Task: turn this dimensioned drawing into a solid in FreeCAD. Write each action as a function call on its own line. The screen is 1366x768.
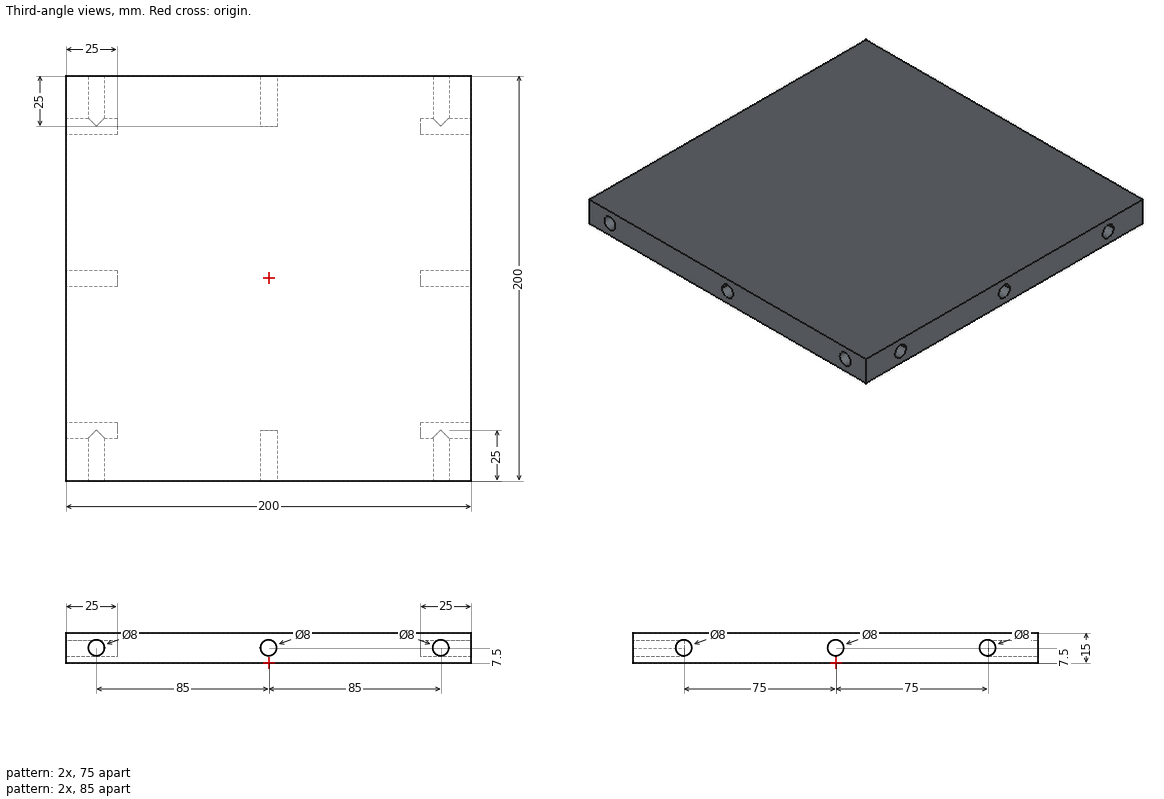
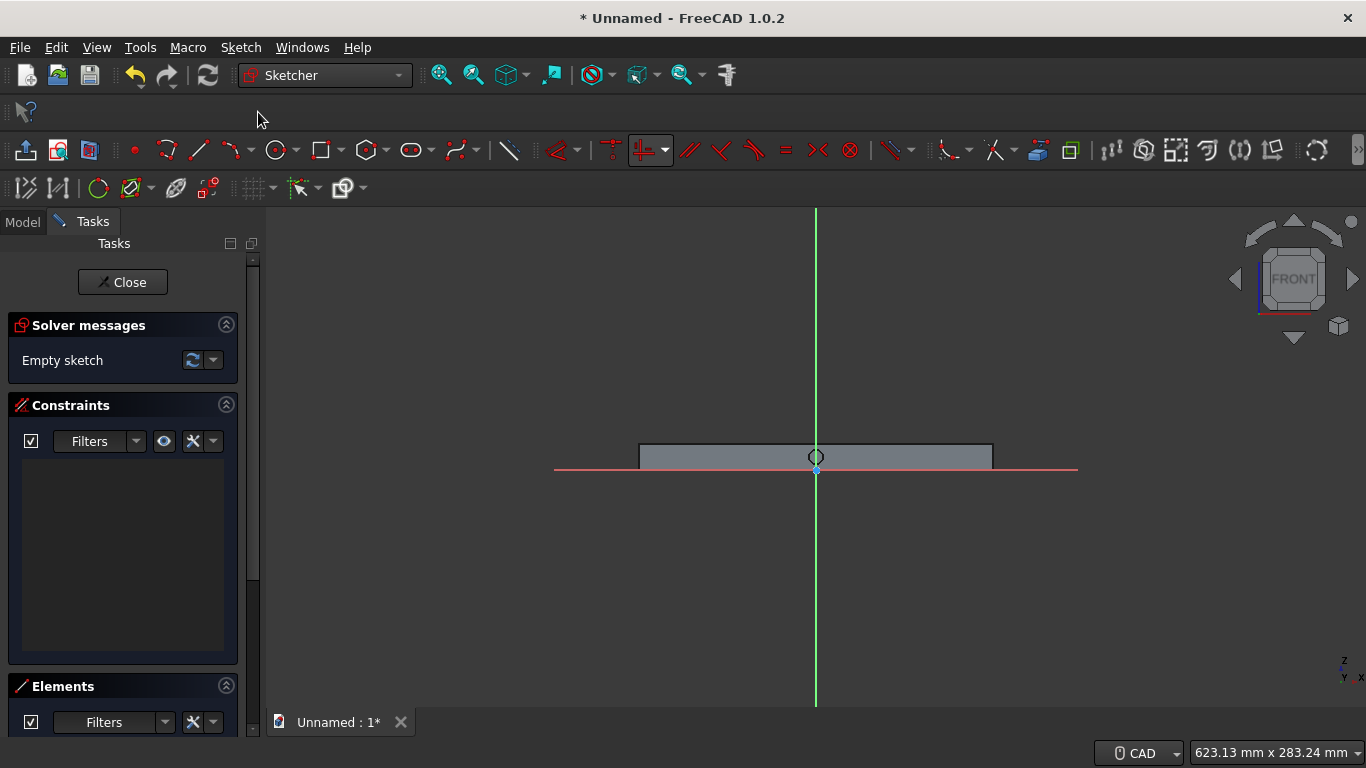
scroll(978, 457, up, 15)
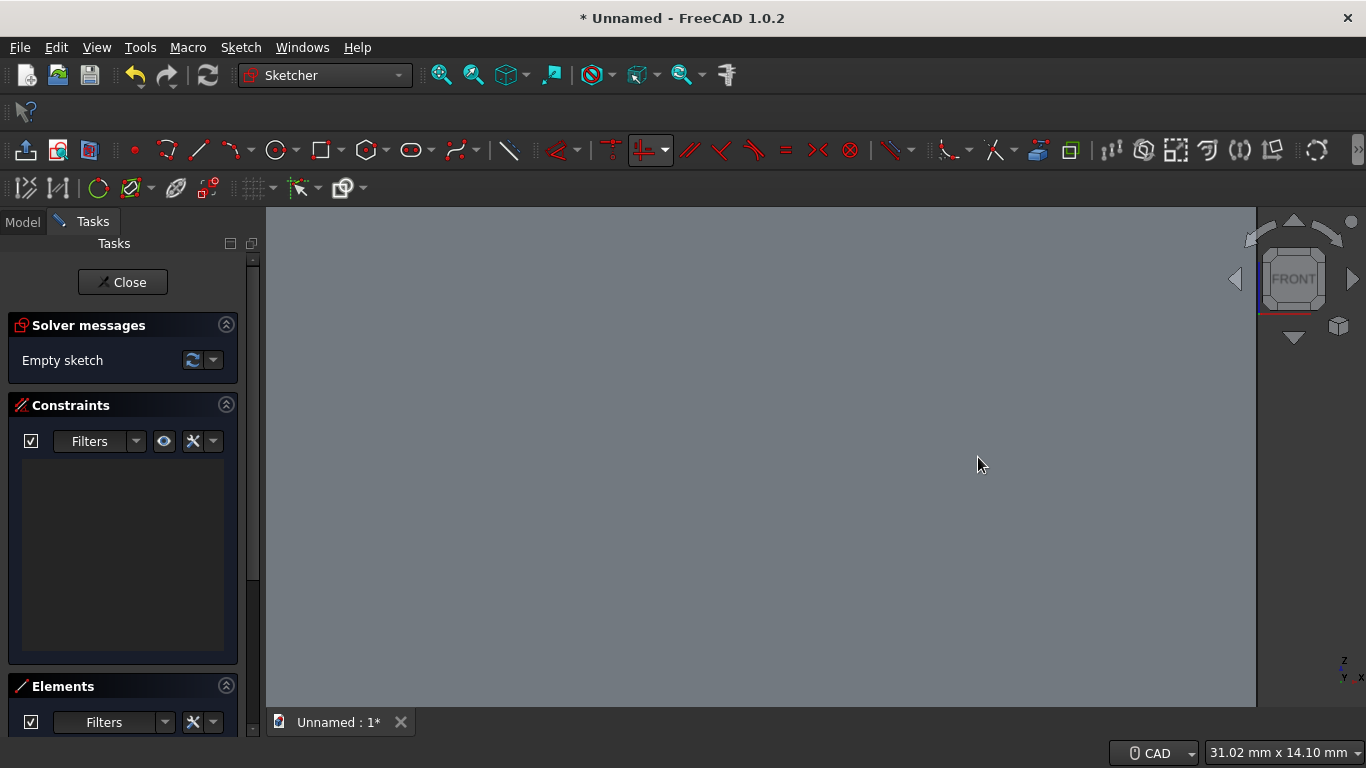
key(g)
key(c)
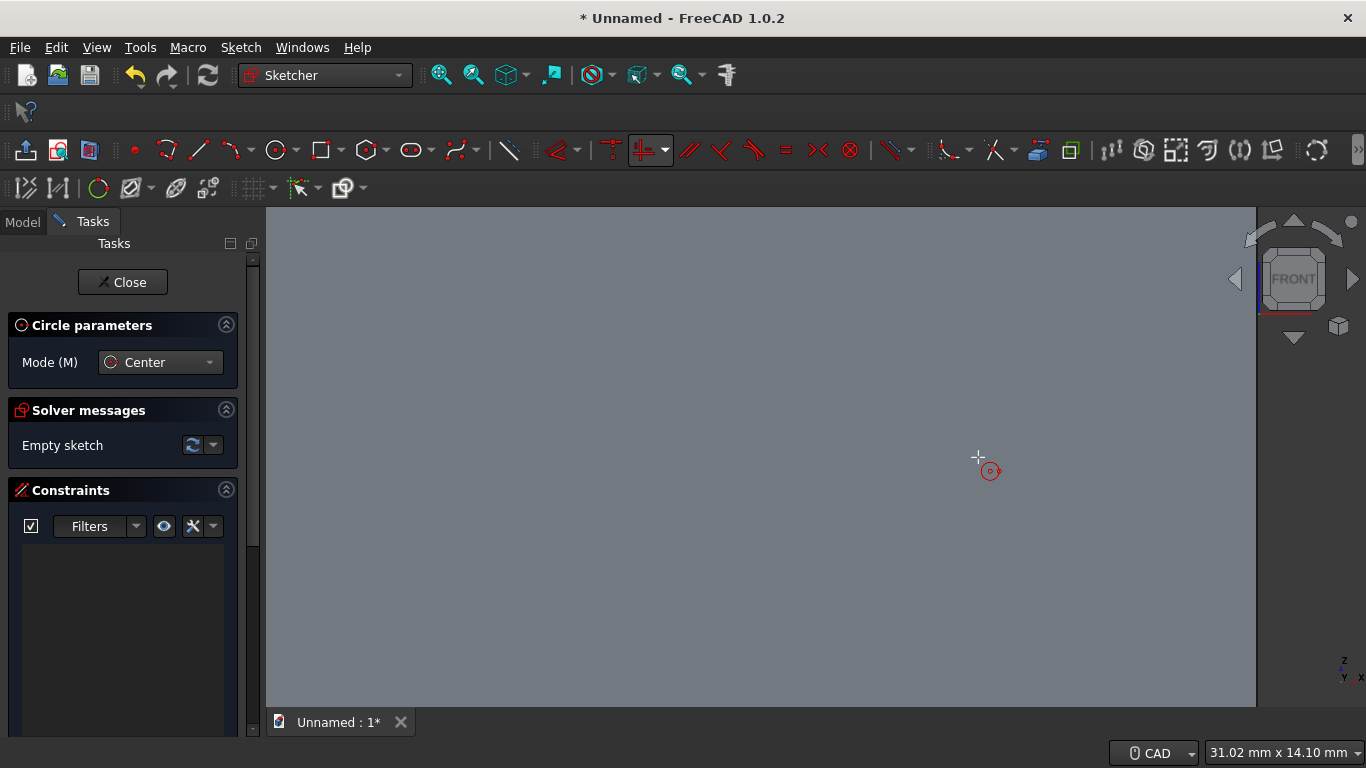
click(726, 447)
move(826, 347)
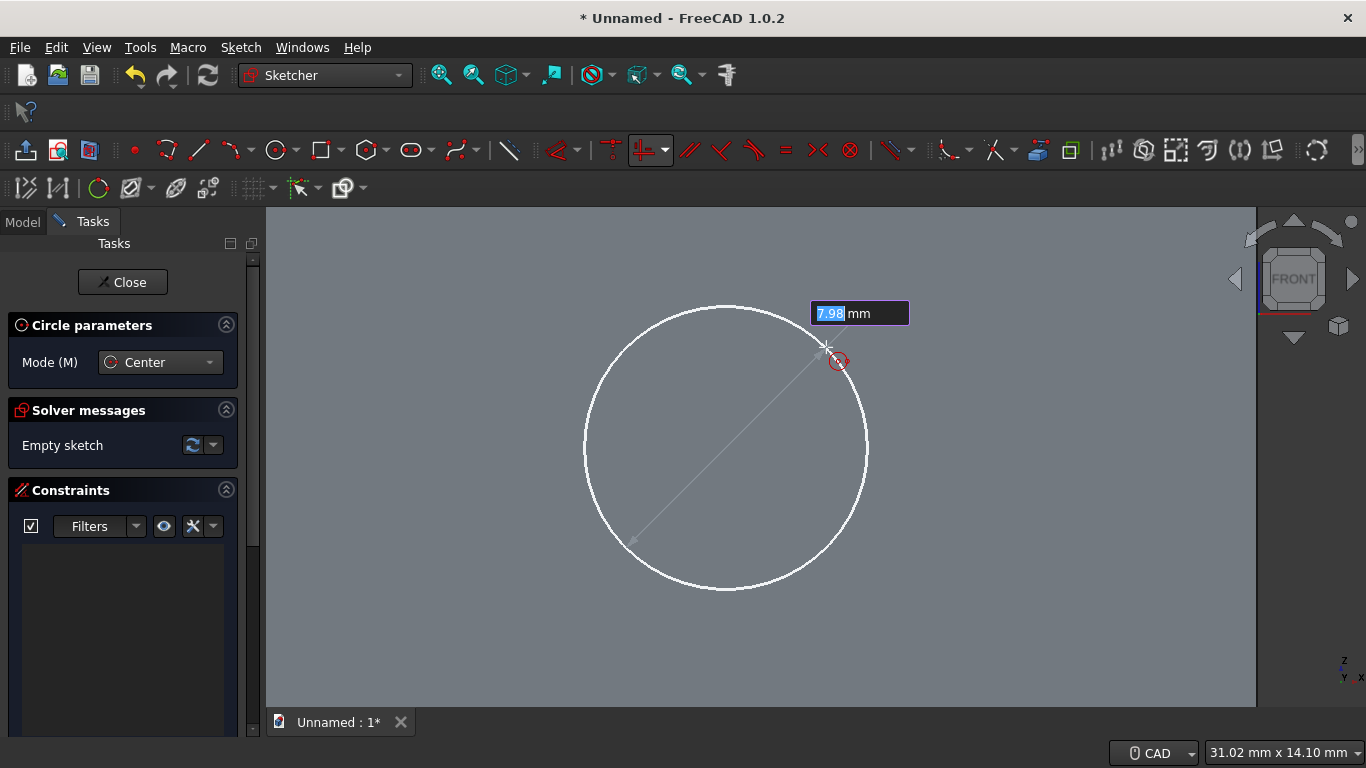
text(8)
key(Return)
key(Escape)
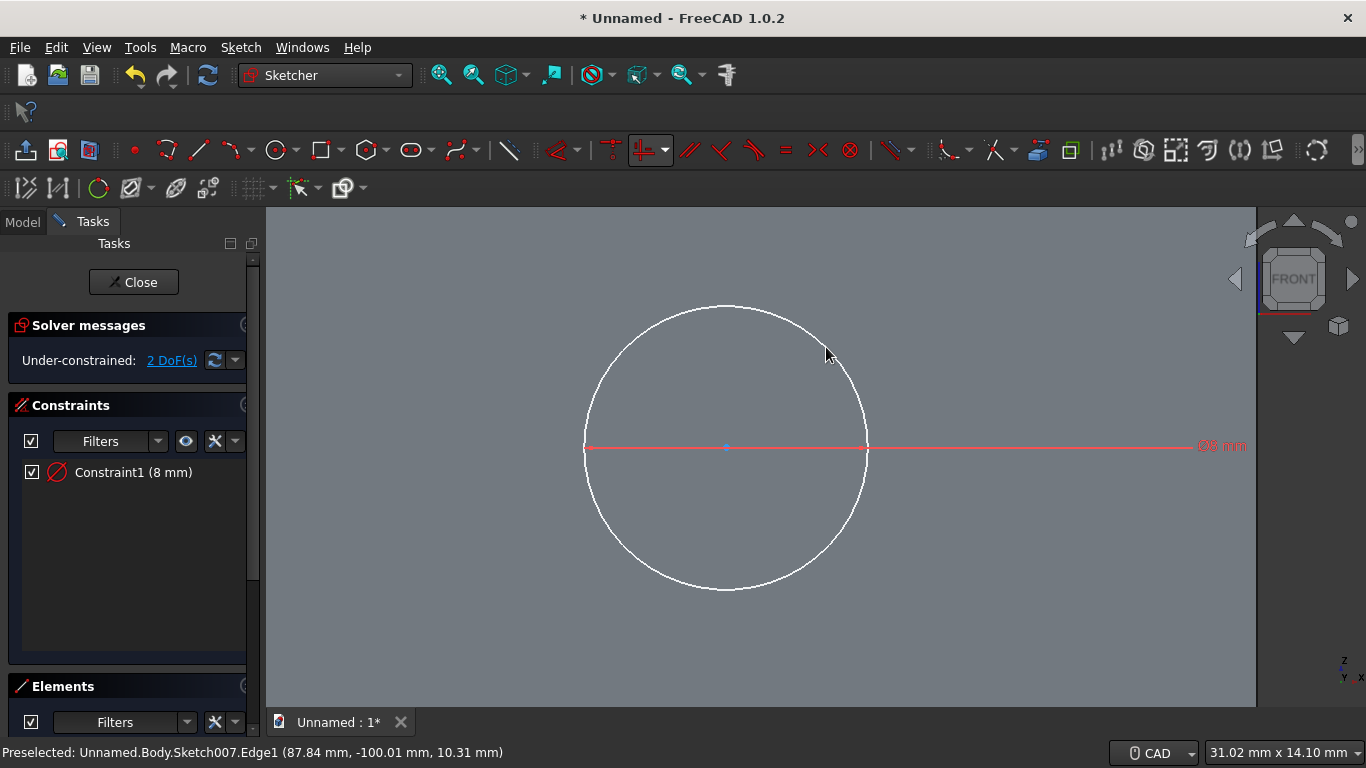
click(556, 150)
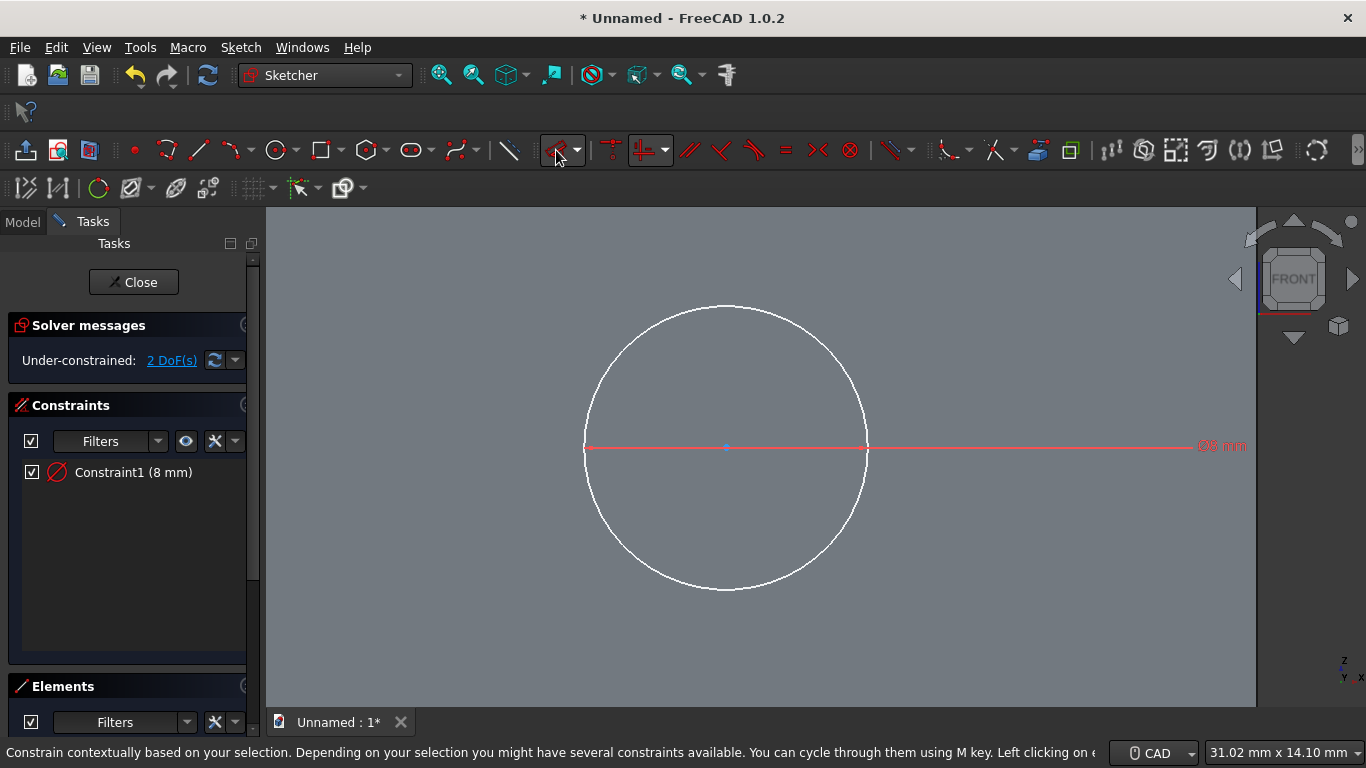
click(726, 448)
click(510, 414)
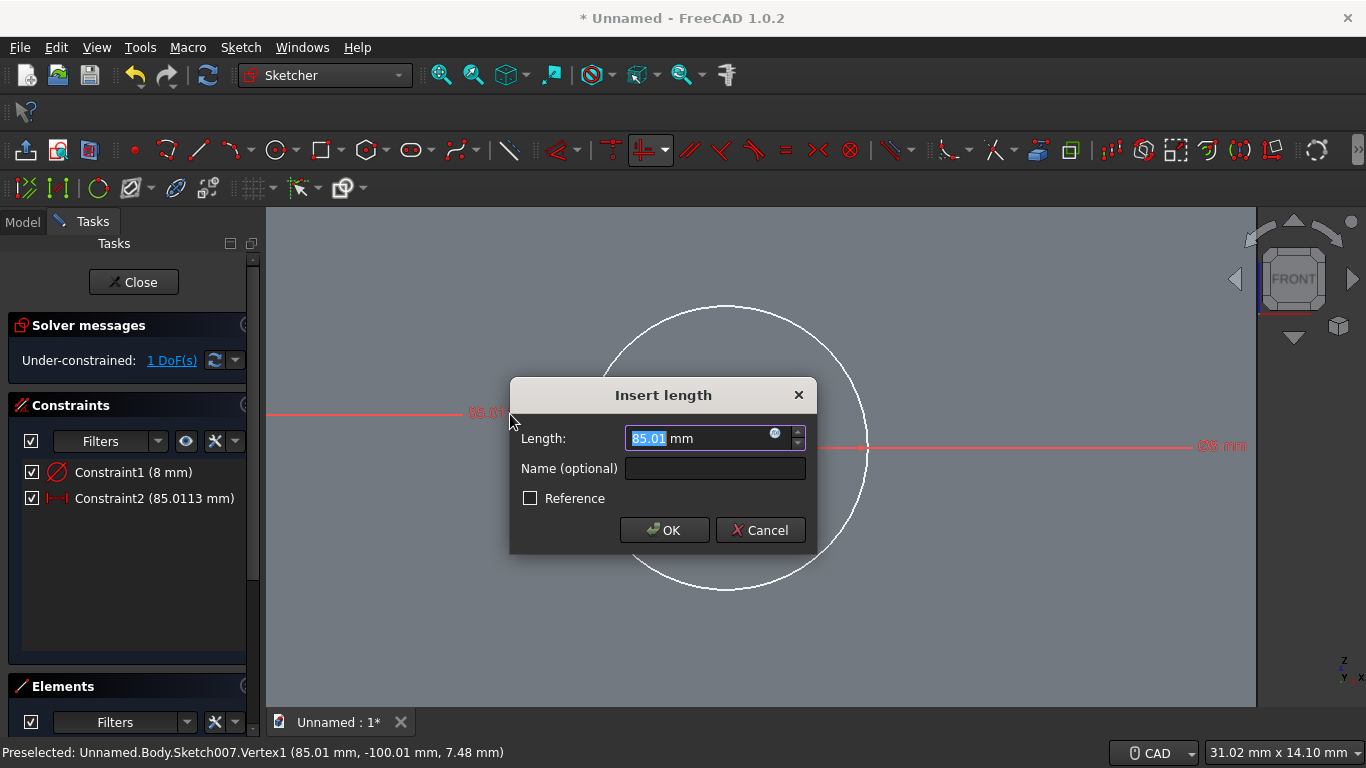
text(85)
key(Return)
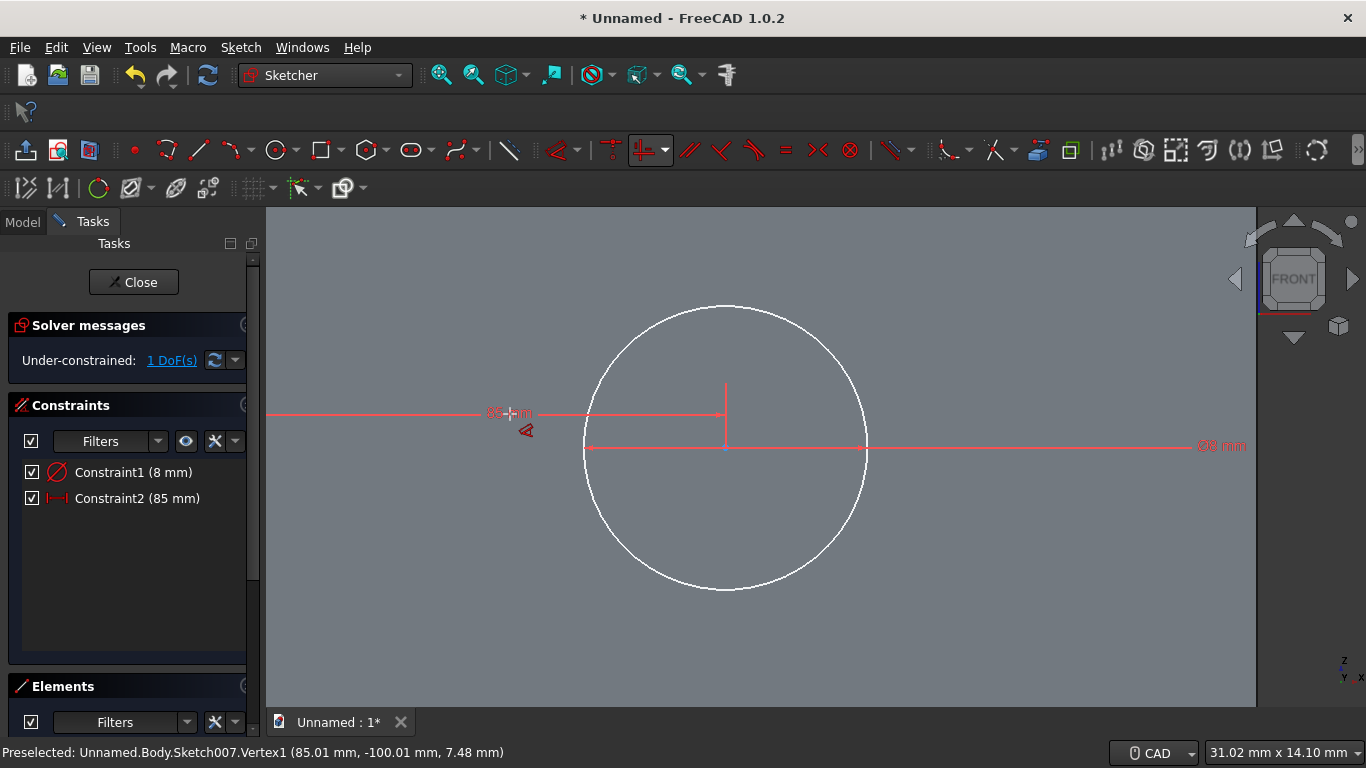
click(726, 448)
click(760, 563)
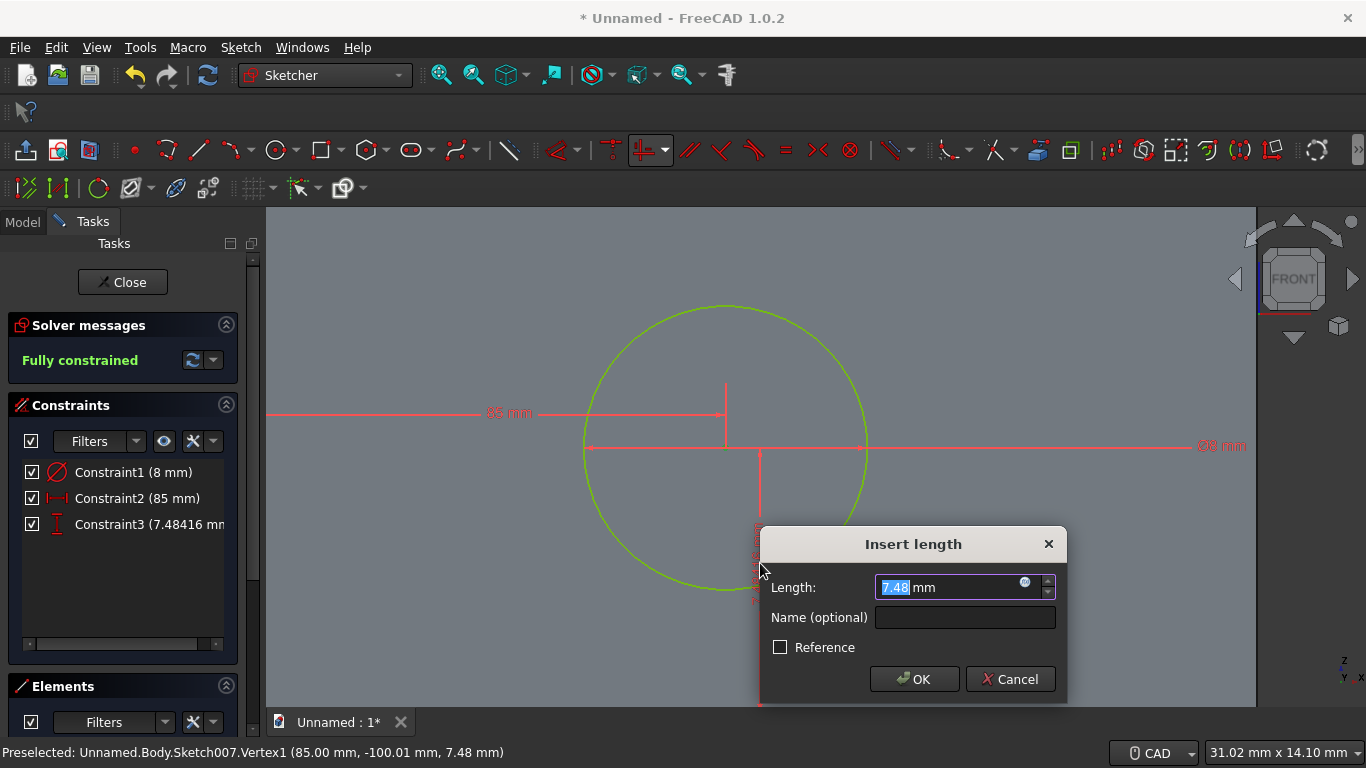
text(7.5)
key(Return)
key(Escape)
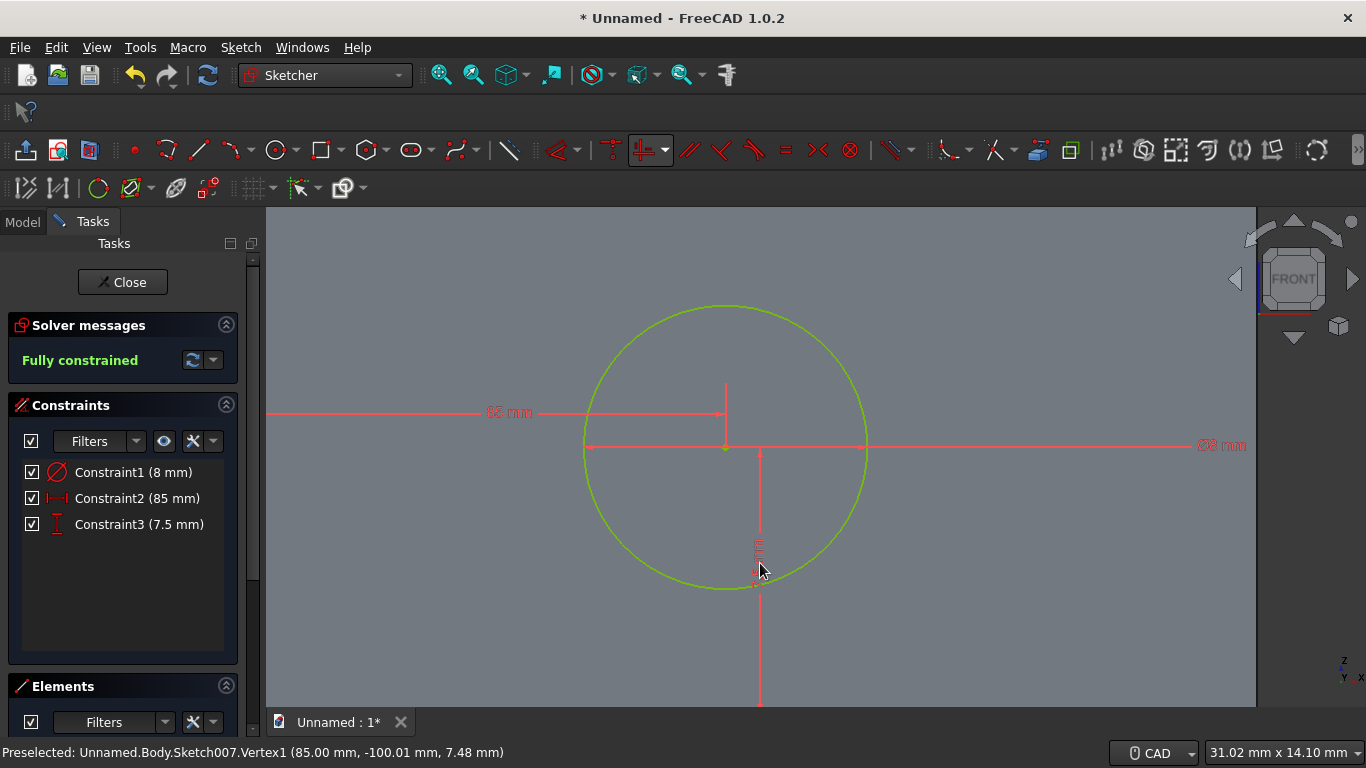
click(123, 282)